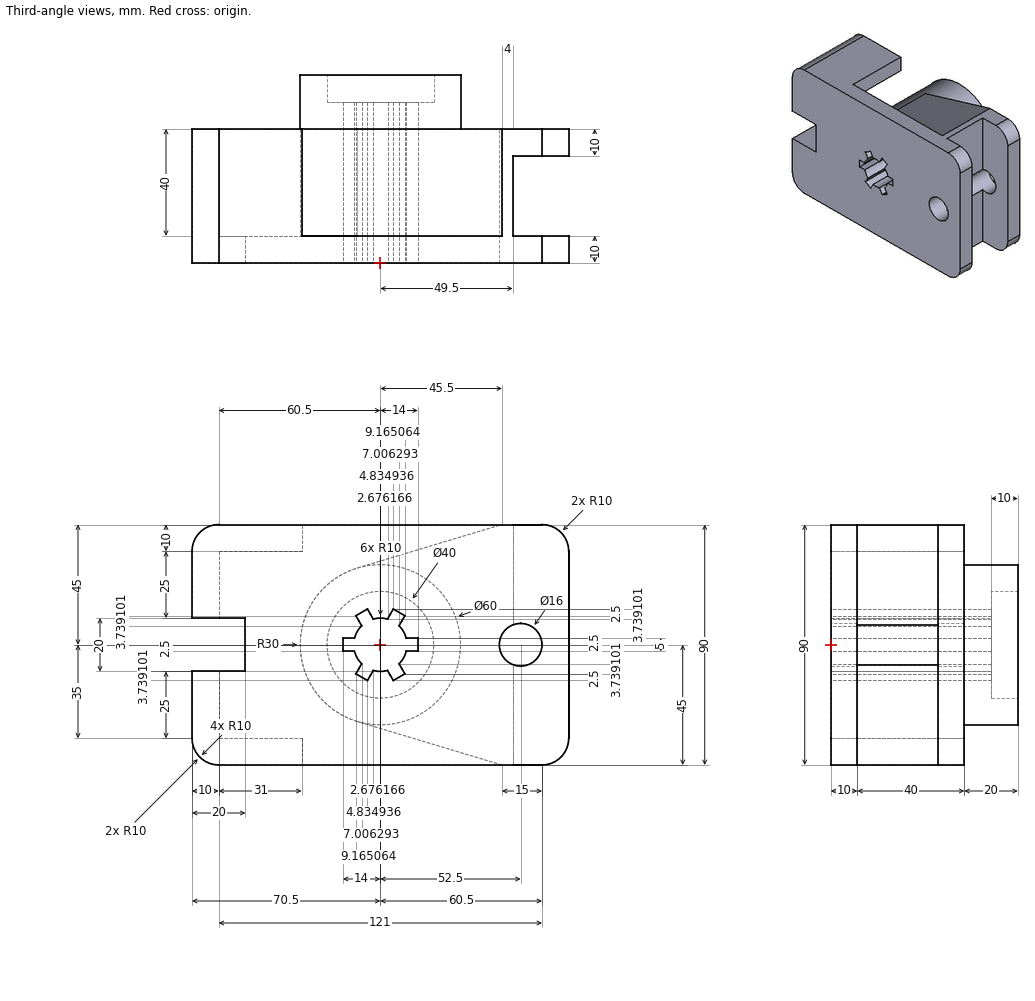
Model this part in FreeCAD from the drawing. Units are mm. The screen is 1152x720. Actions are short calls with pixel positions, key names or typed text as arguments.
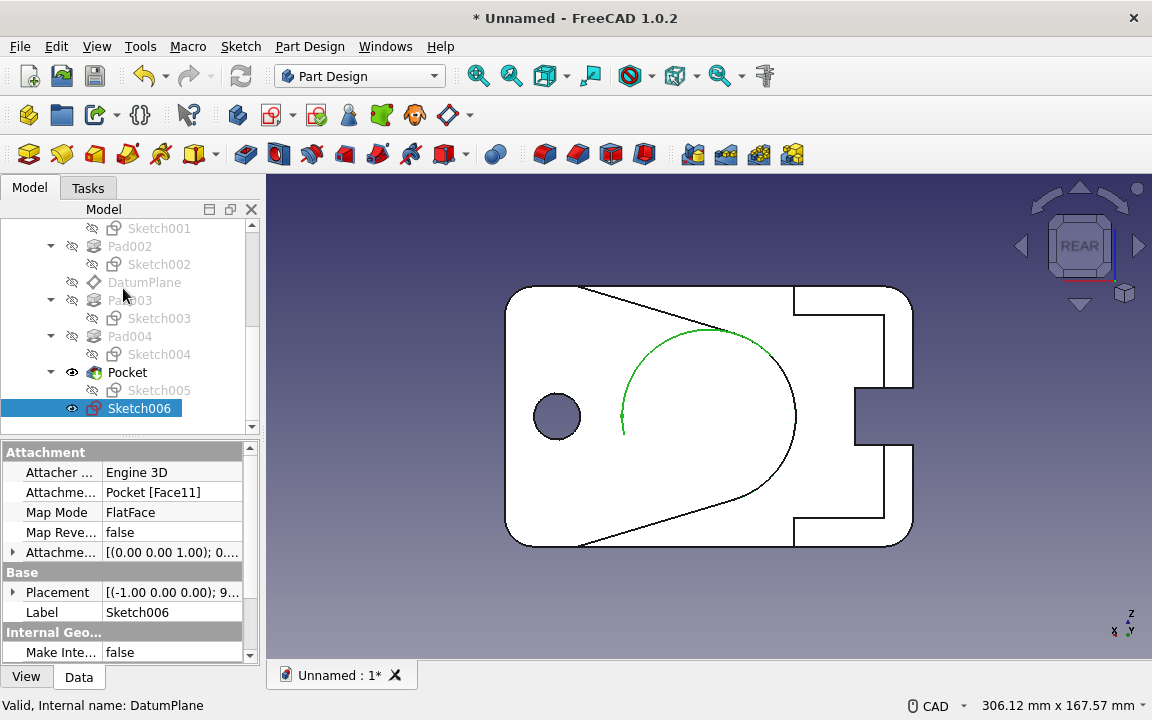
click(29, 154)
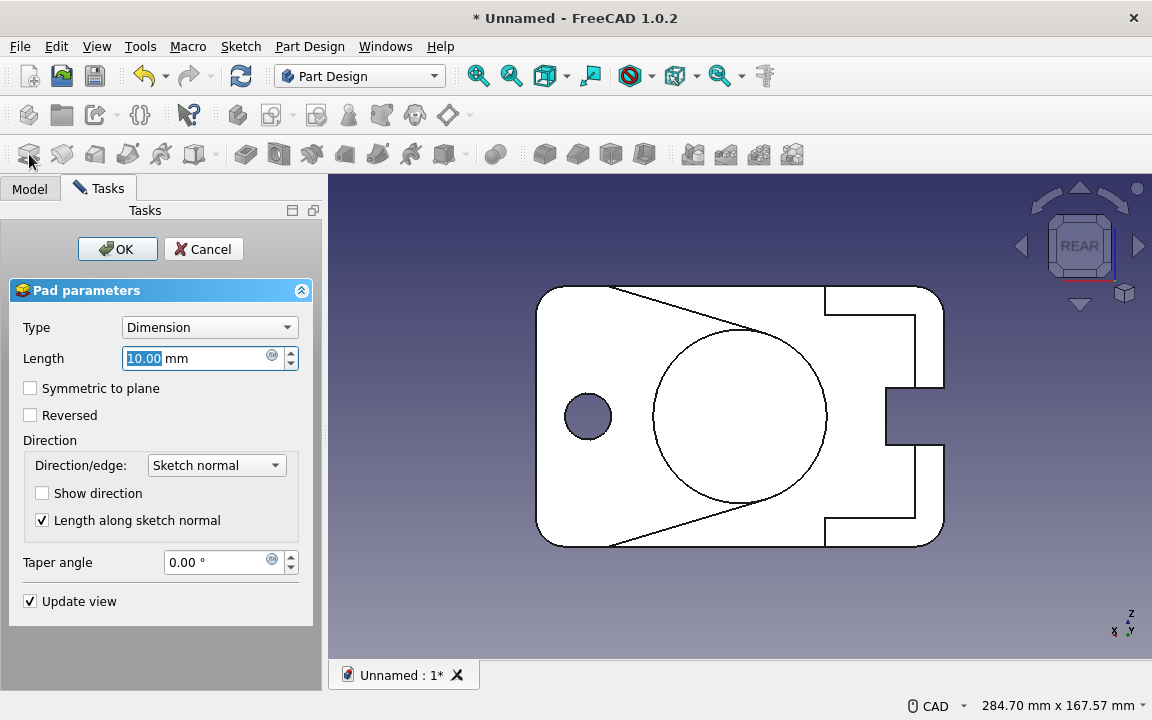
text(20)
key(Tab)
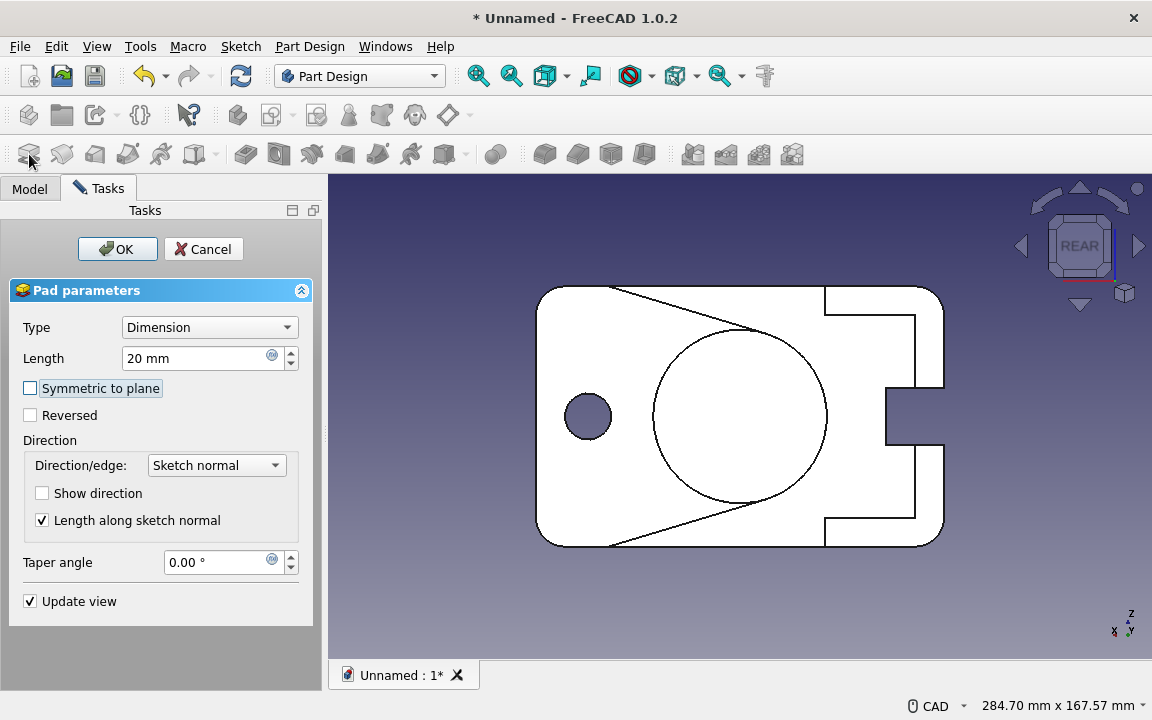
click(118, 249)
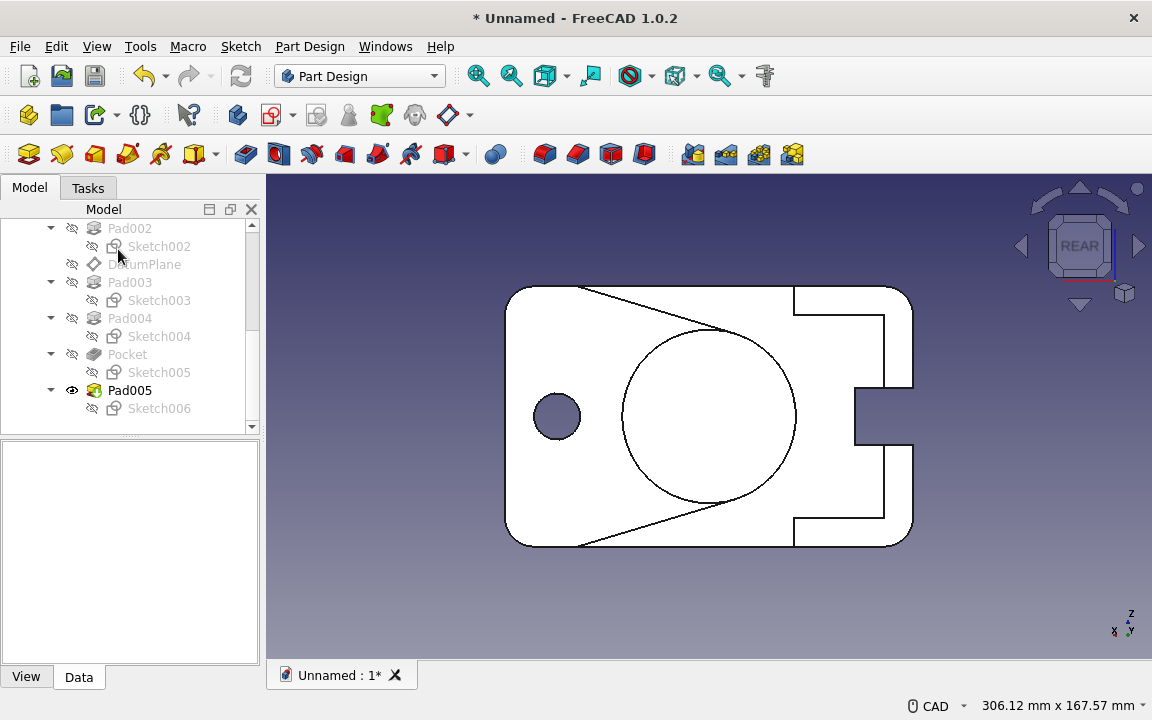
click(709, 416)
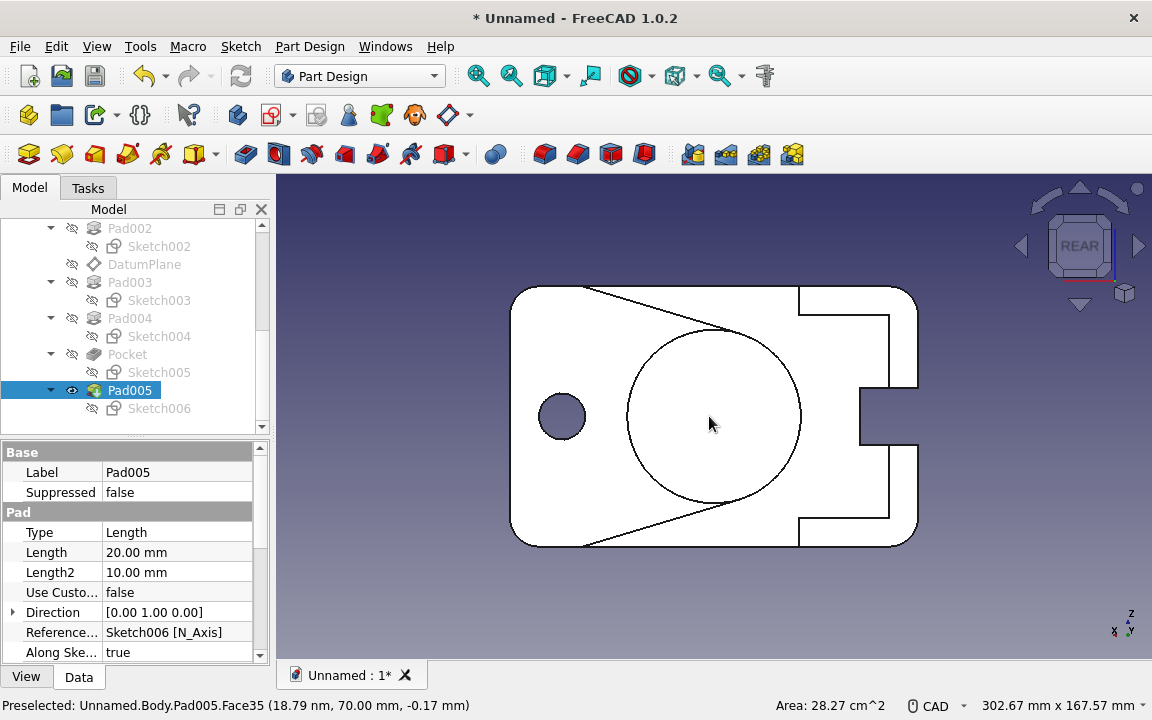
click(270, 116)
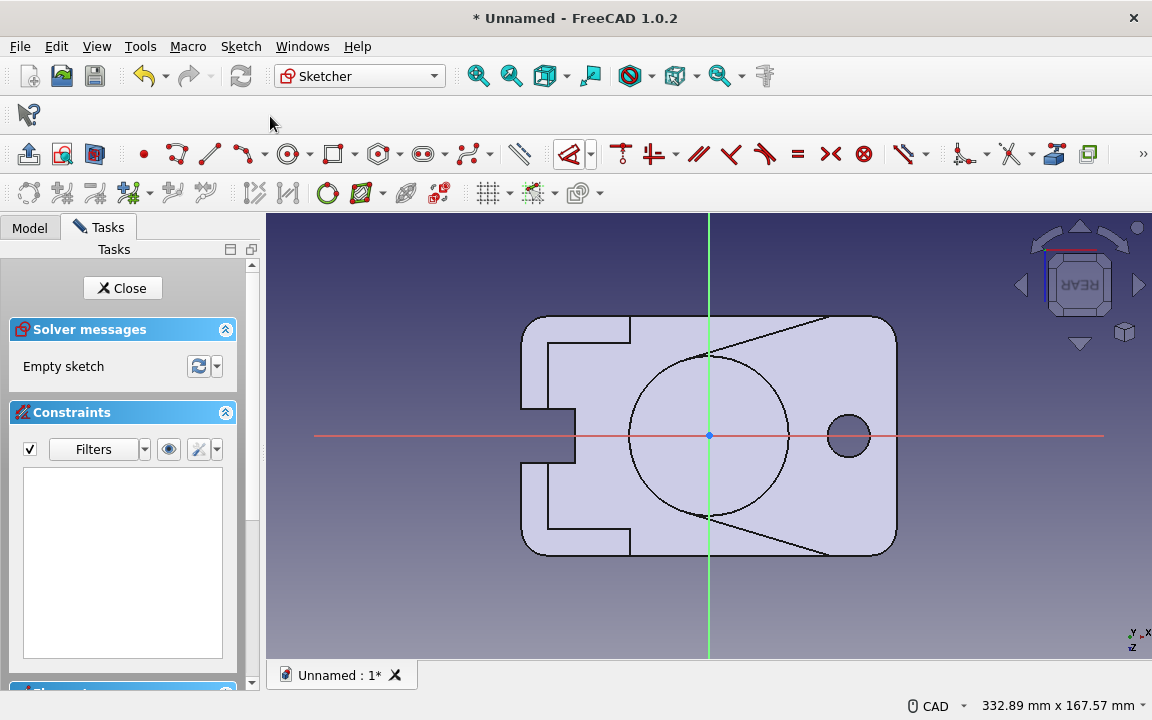
scroll(749, 436, up, 5)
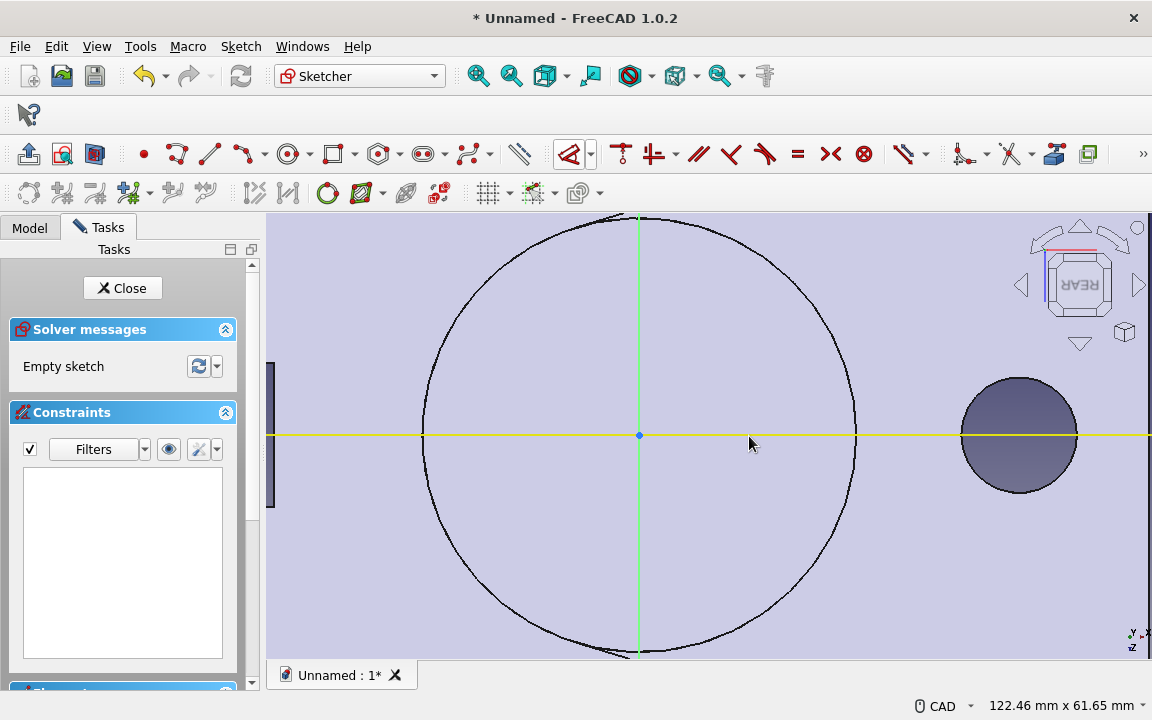
click(288, 154)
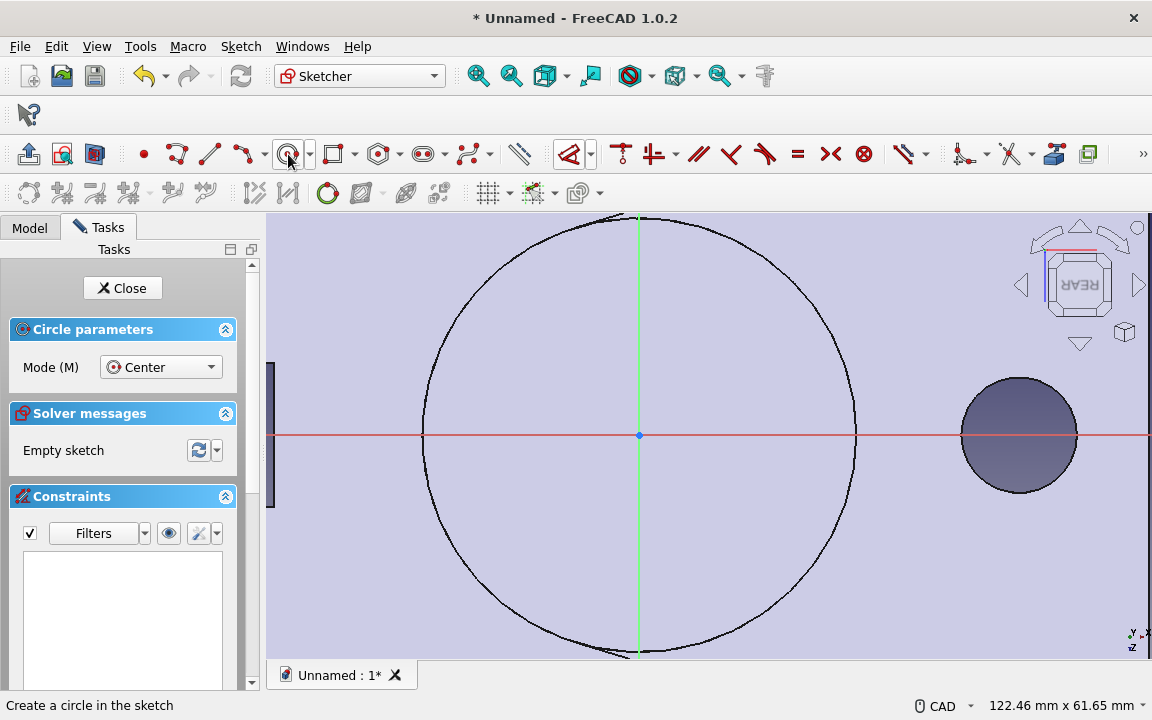
click(639, 435)
move(742, 333)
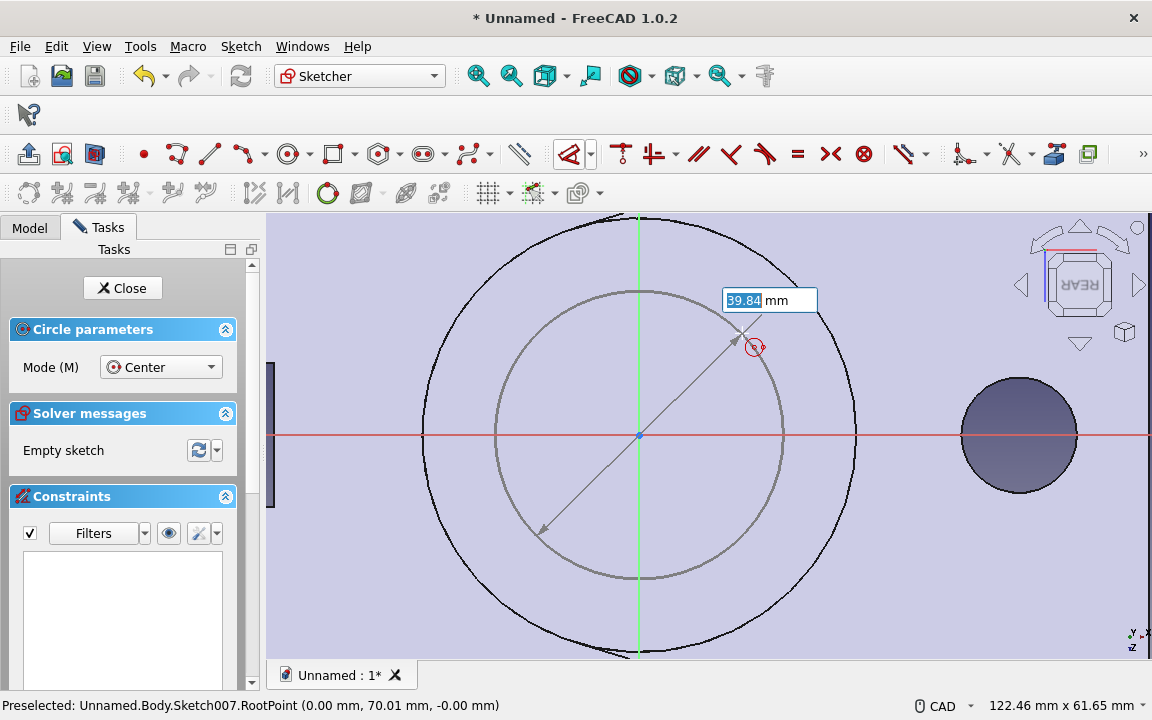
text(40)
key(Return)
key(Escape)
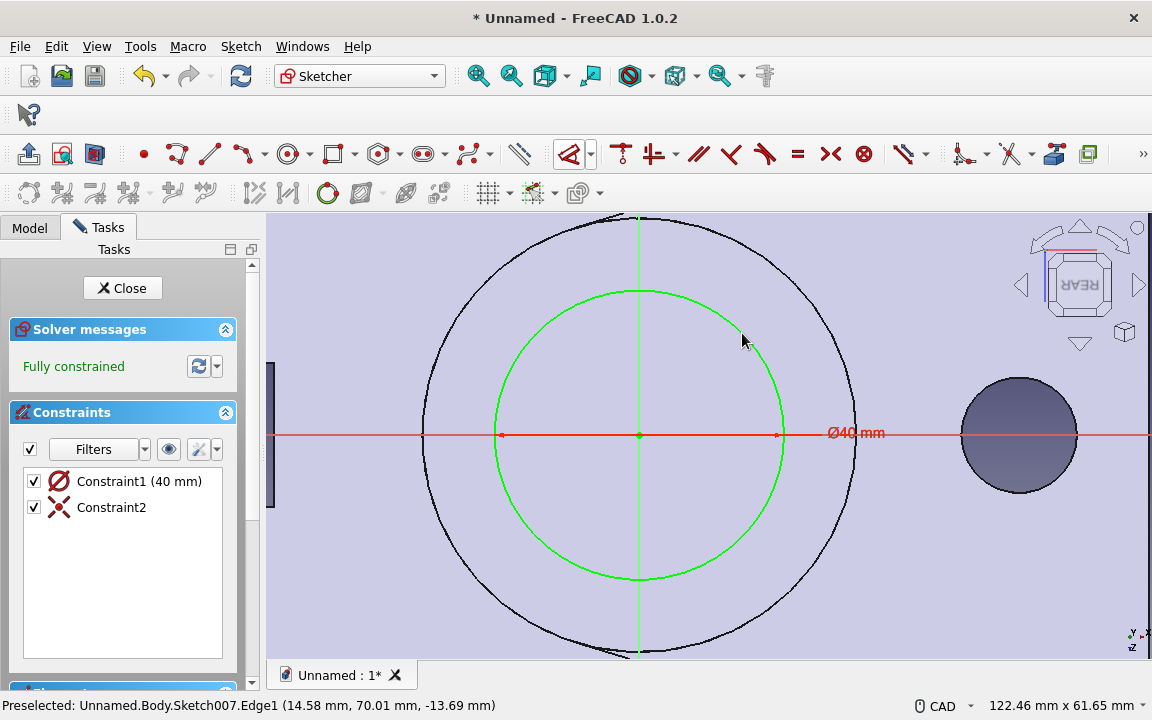
click(123, 288)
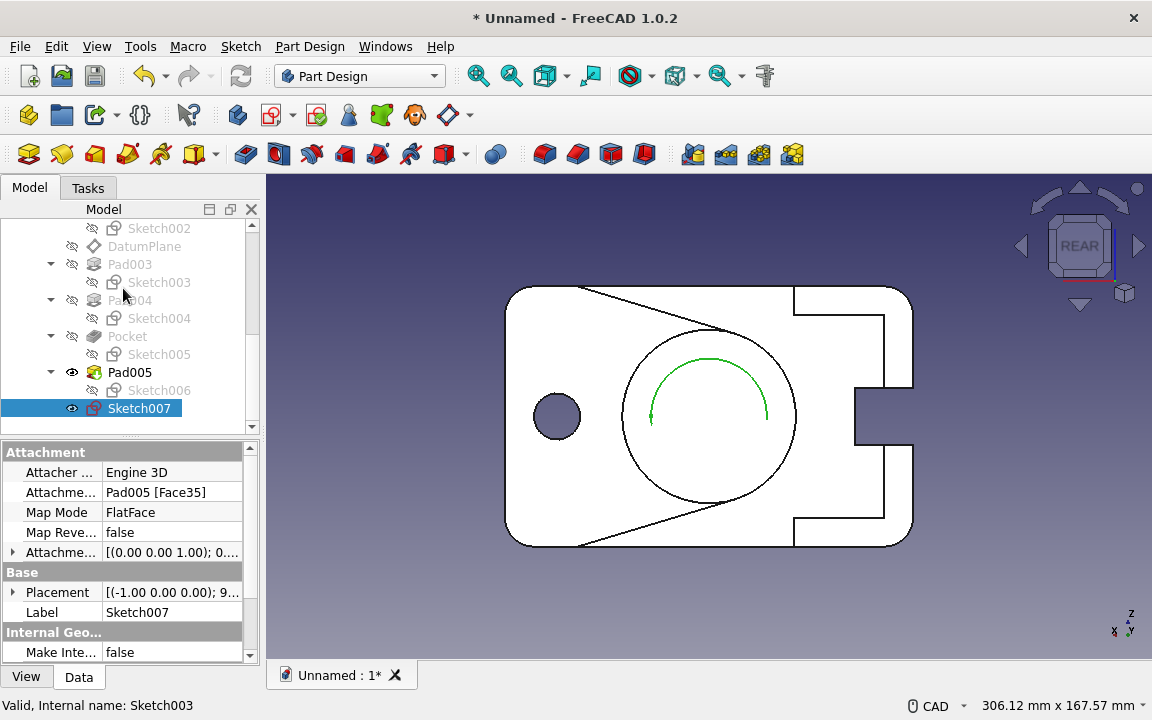
click(246, 154)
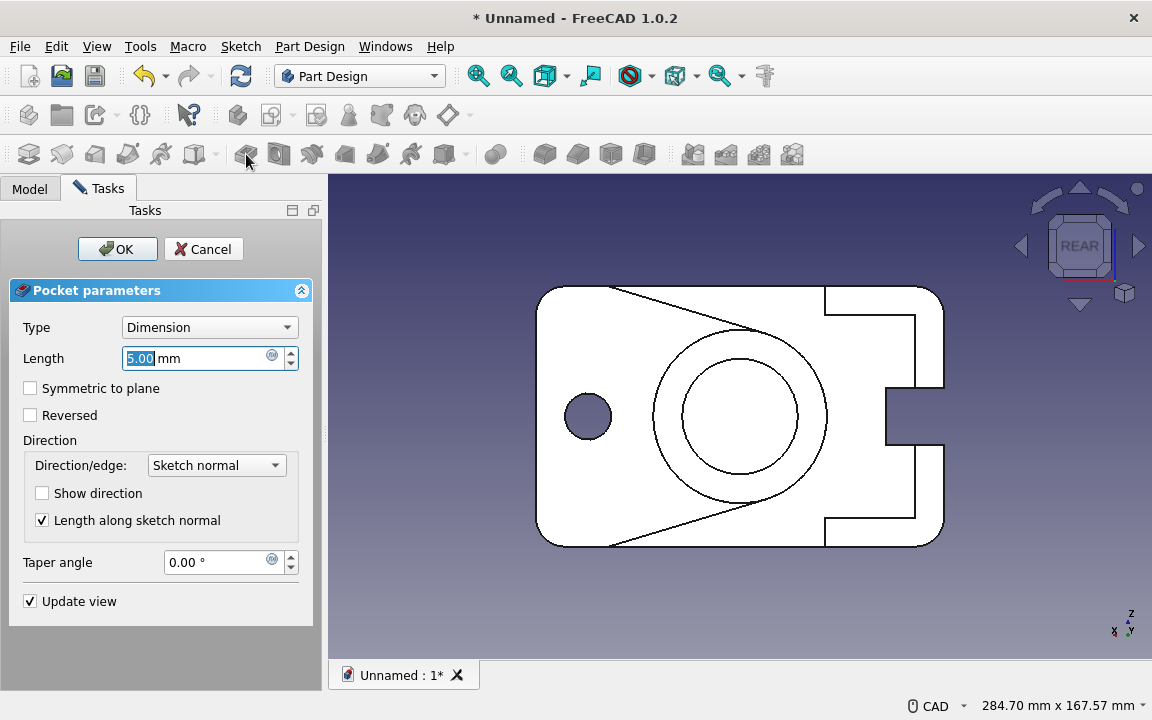
text(10)
key(Tab)